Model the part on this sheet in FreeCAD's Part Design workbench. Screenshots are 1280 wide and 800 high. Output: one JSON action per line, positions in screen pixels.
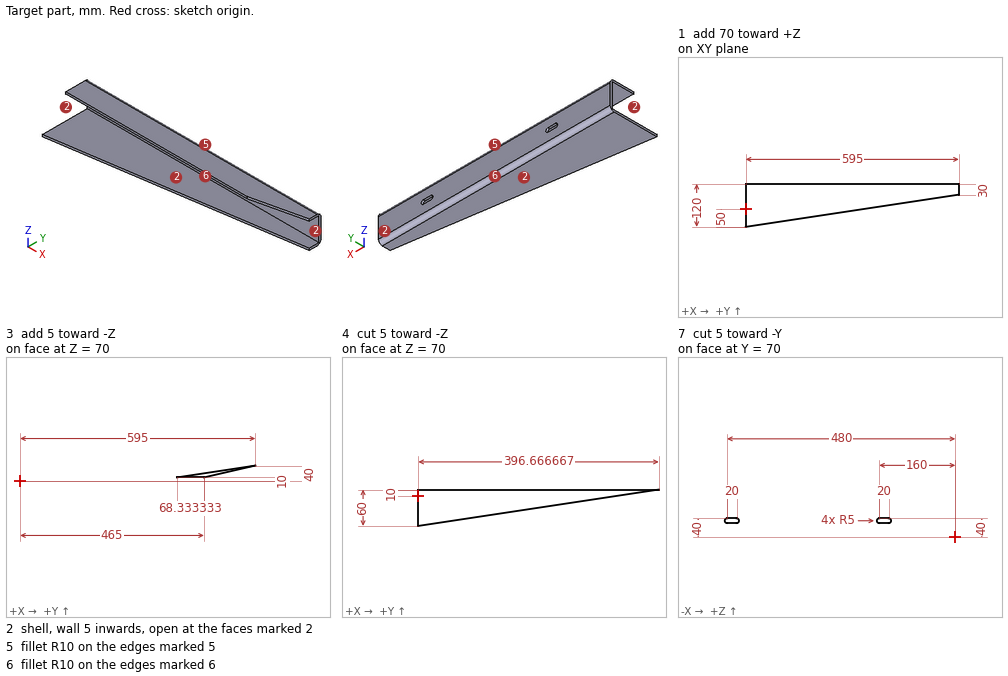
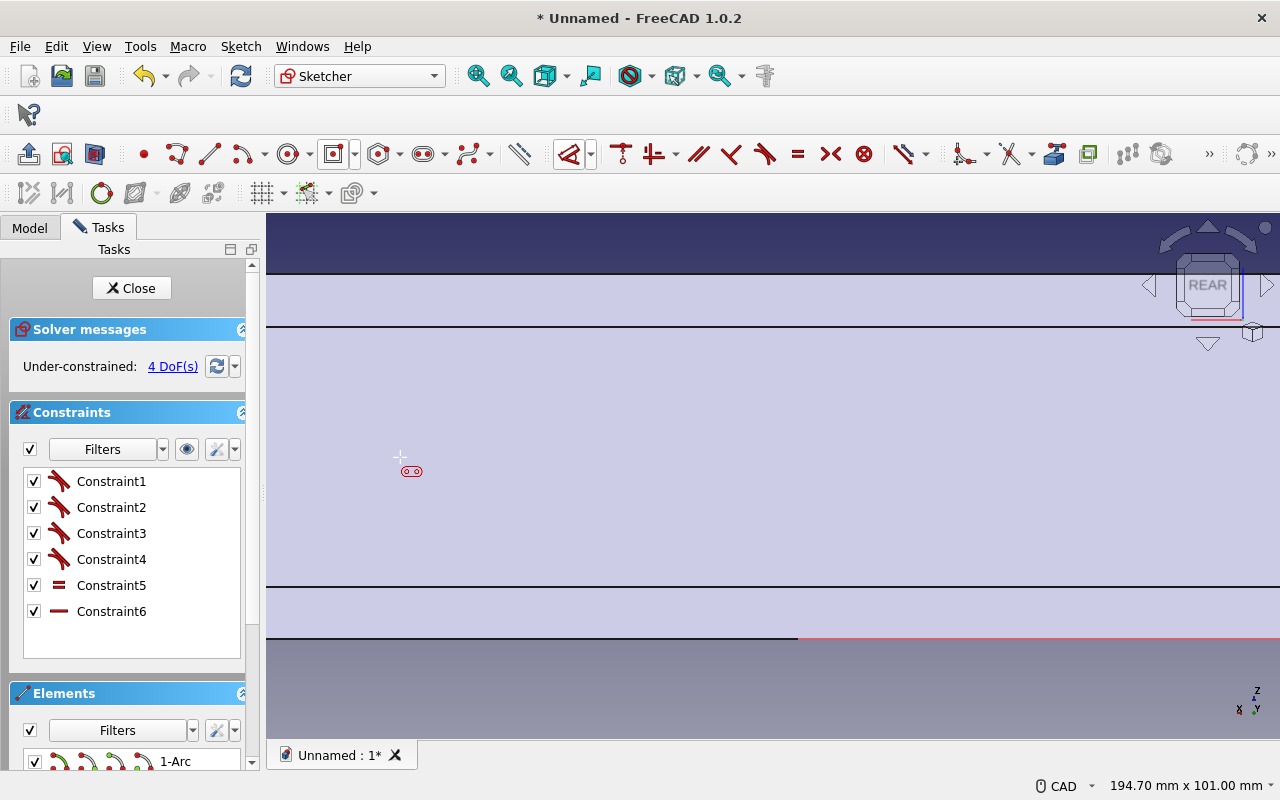
{"action": "scroll", "coordinate": [400, 457], "scroll_direction": "down", "scroll_amount": 7}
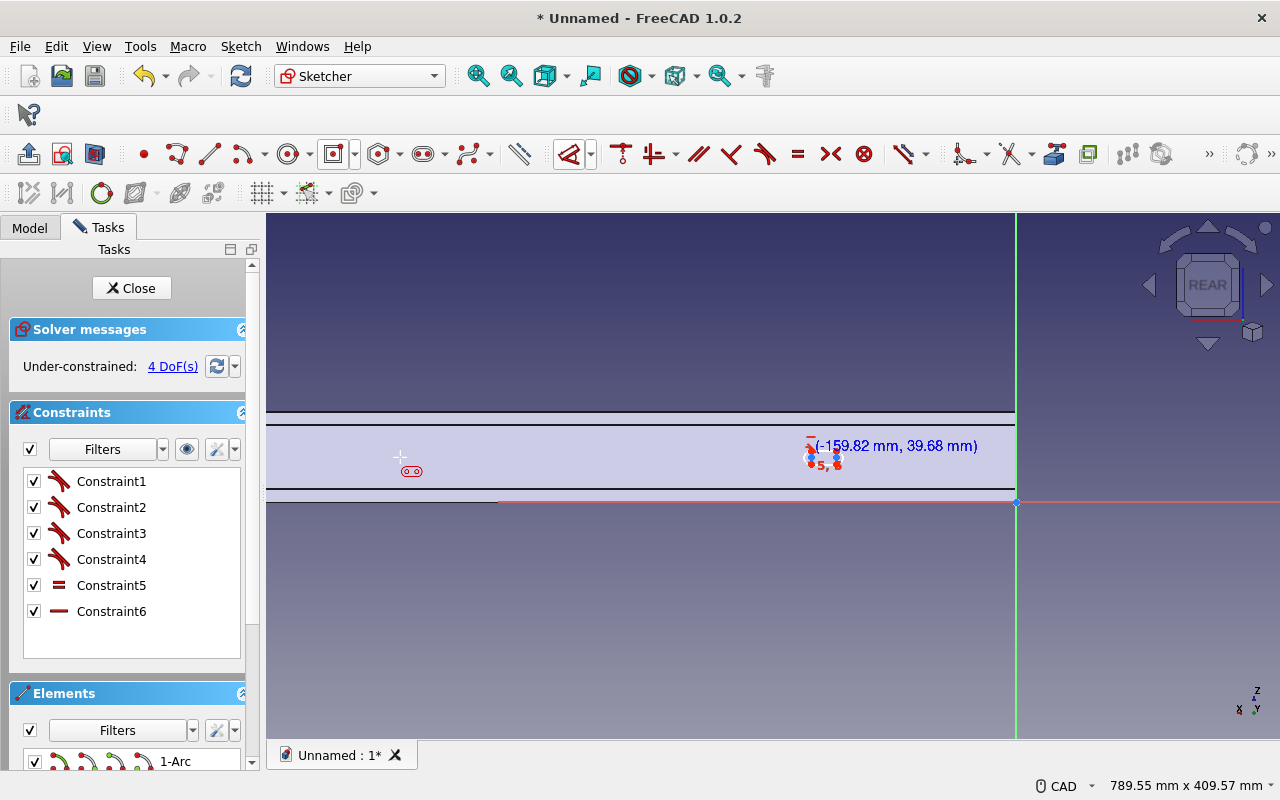
{"action": "left_click", "coordinate": [400, 457]}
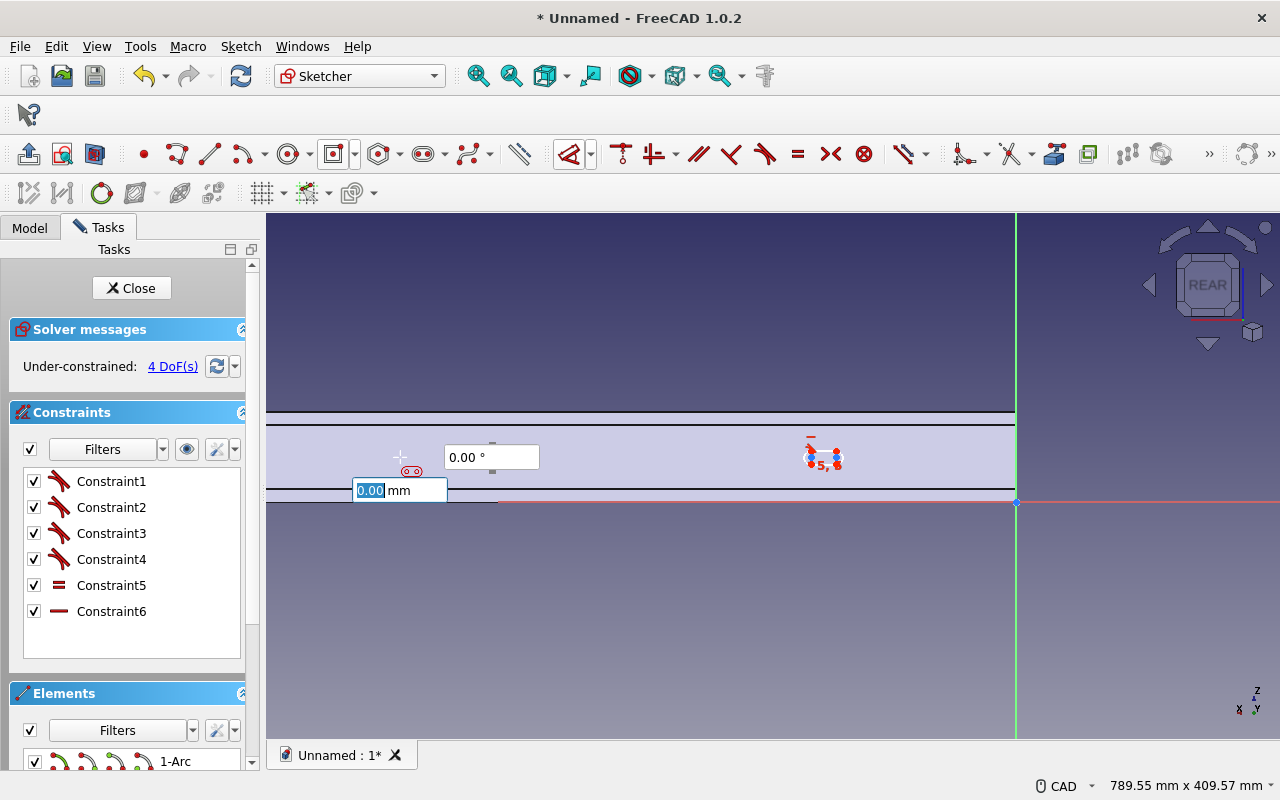
{"action": "left_click", "coordinate": [425, 457]}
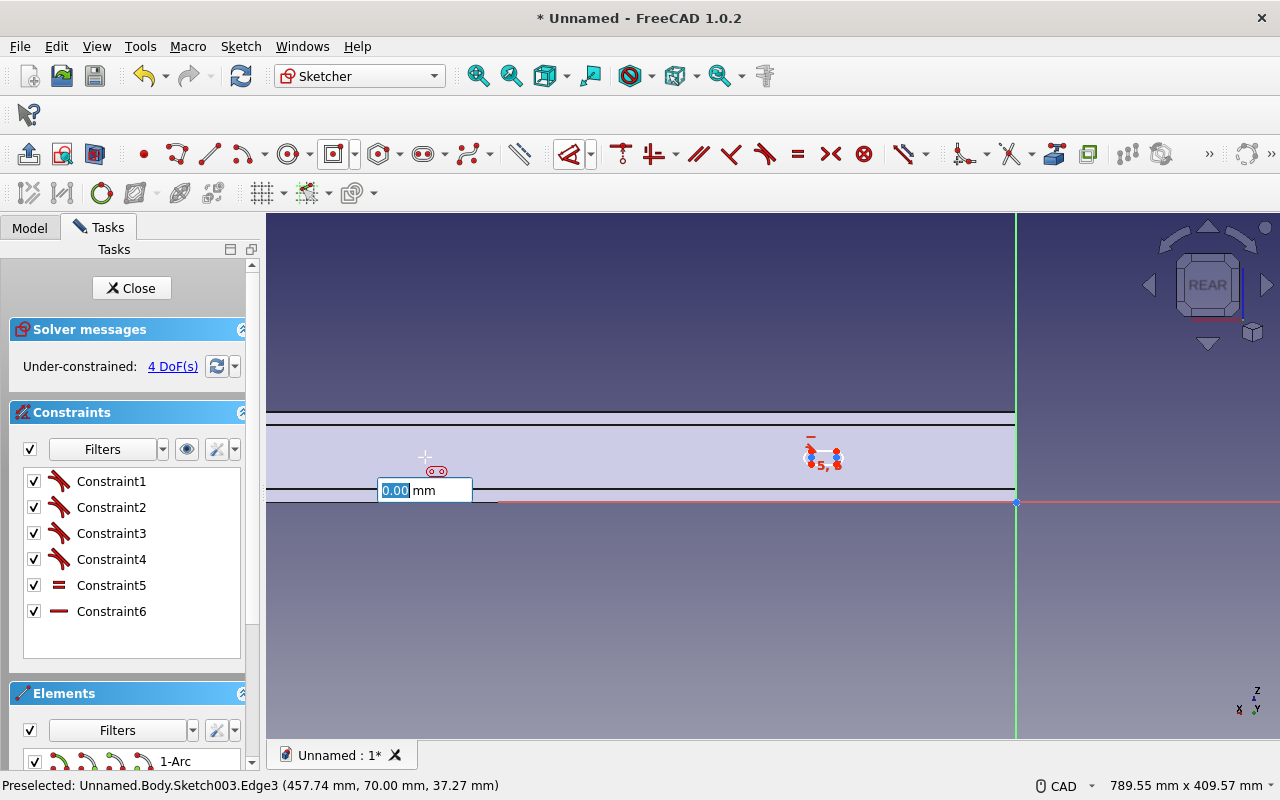
{"action": "scroll", "coordinate": [413, 464], "scroll_direction": "up", "scroll_amount": 5}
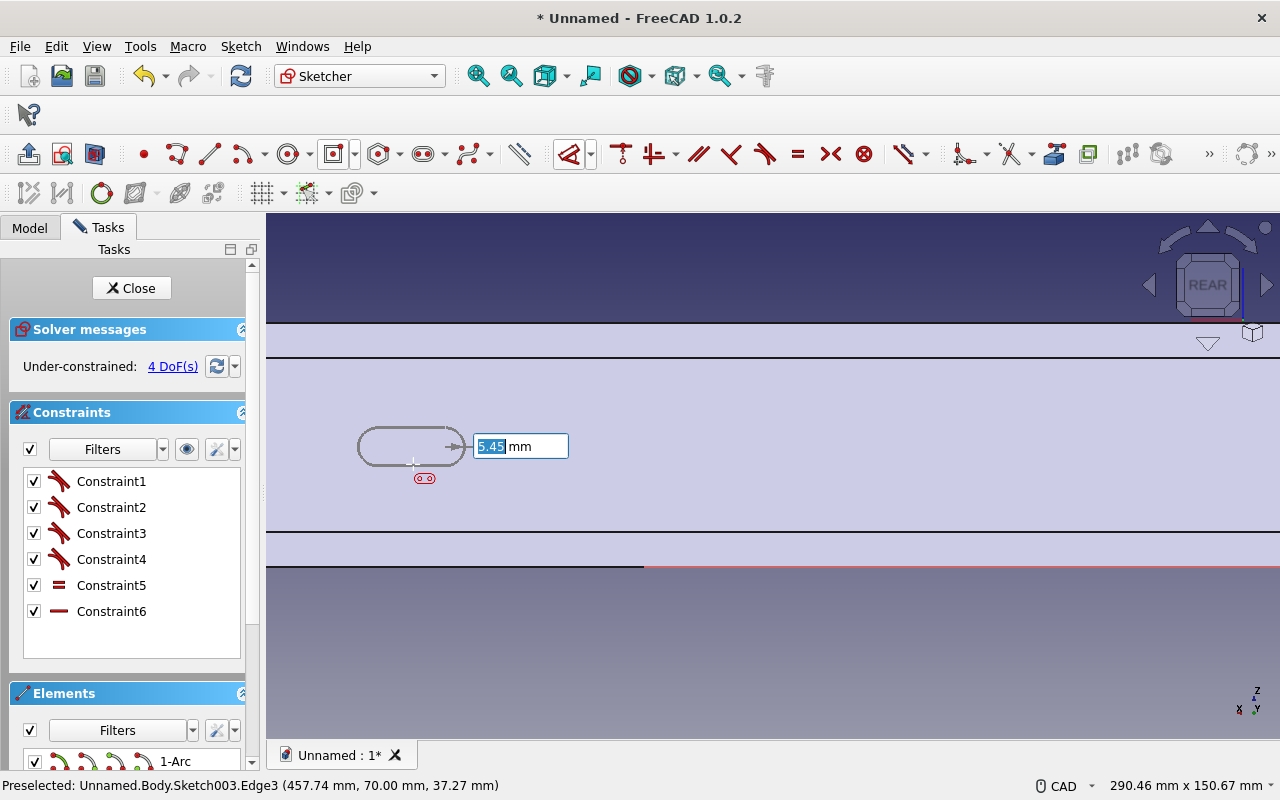
{"action": "left_click", "coordinate": [412, 462]}
{"action": "key", "text": "Escape"}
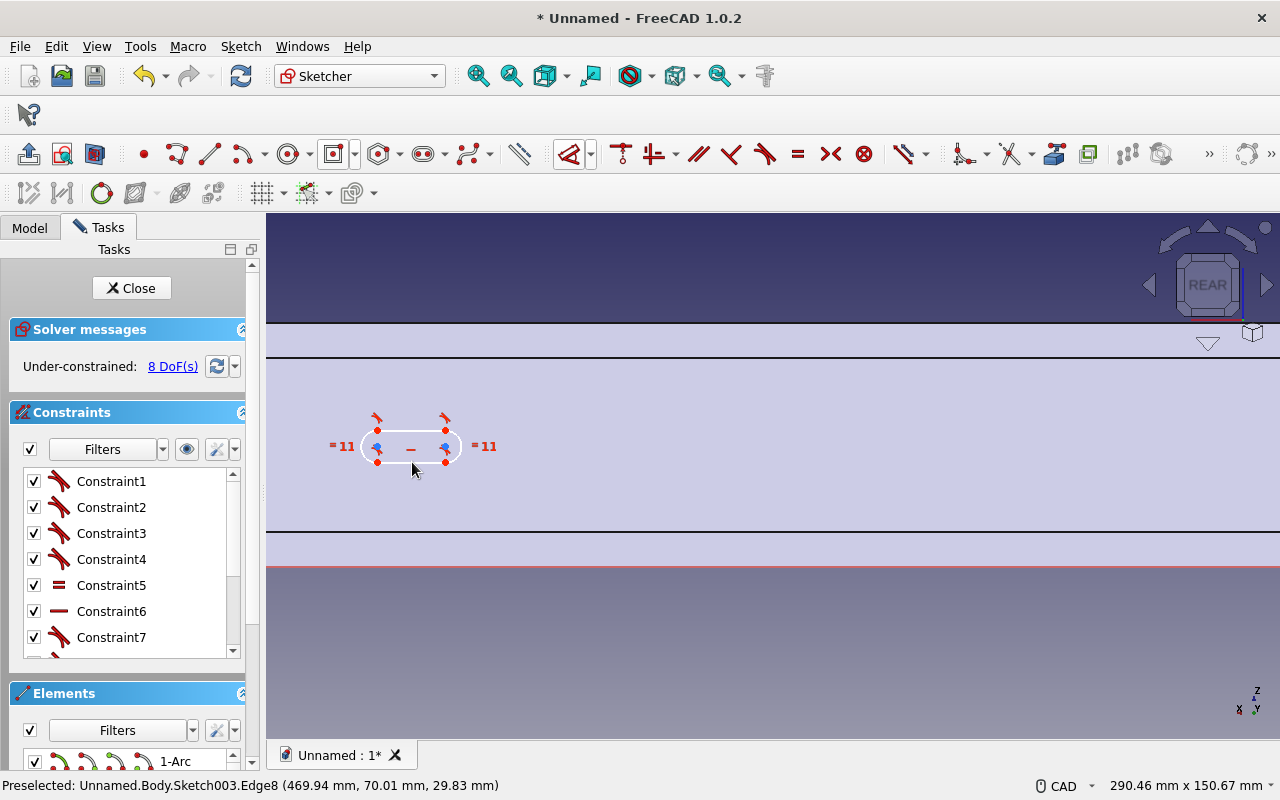
{"action": "scroll", "coordinate": [413, 464], "scroll_direction": "down", "scroll_amount": 5}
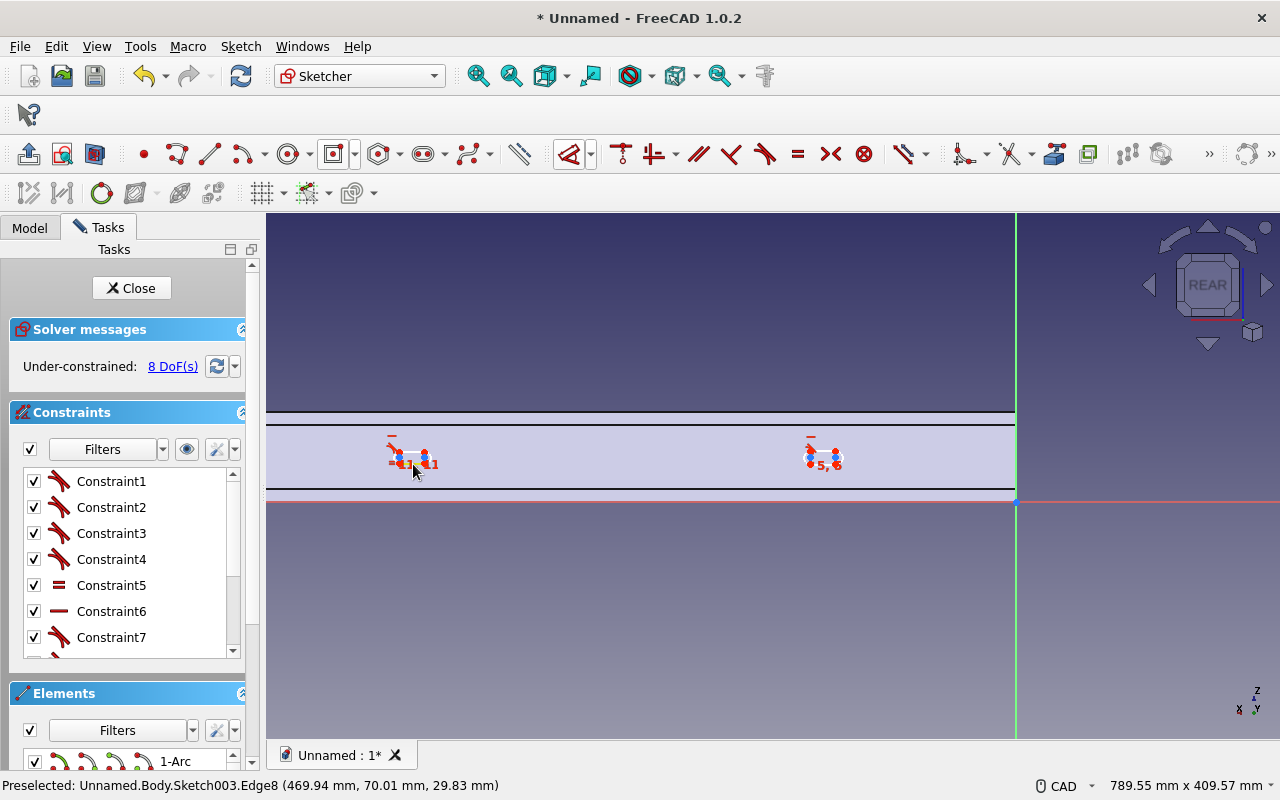
{"action": "scroll", "coordinate": [806, 454], "scroll_direction": "up", "scroll_amount": 5}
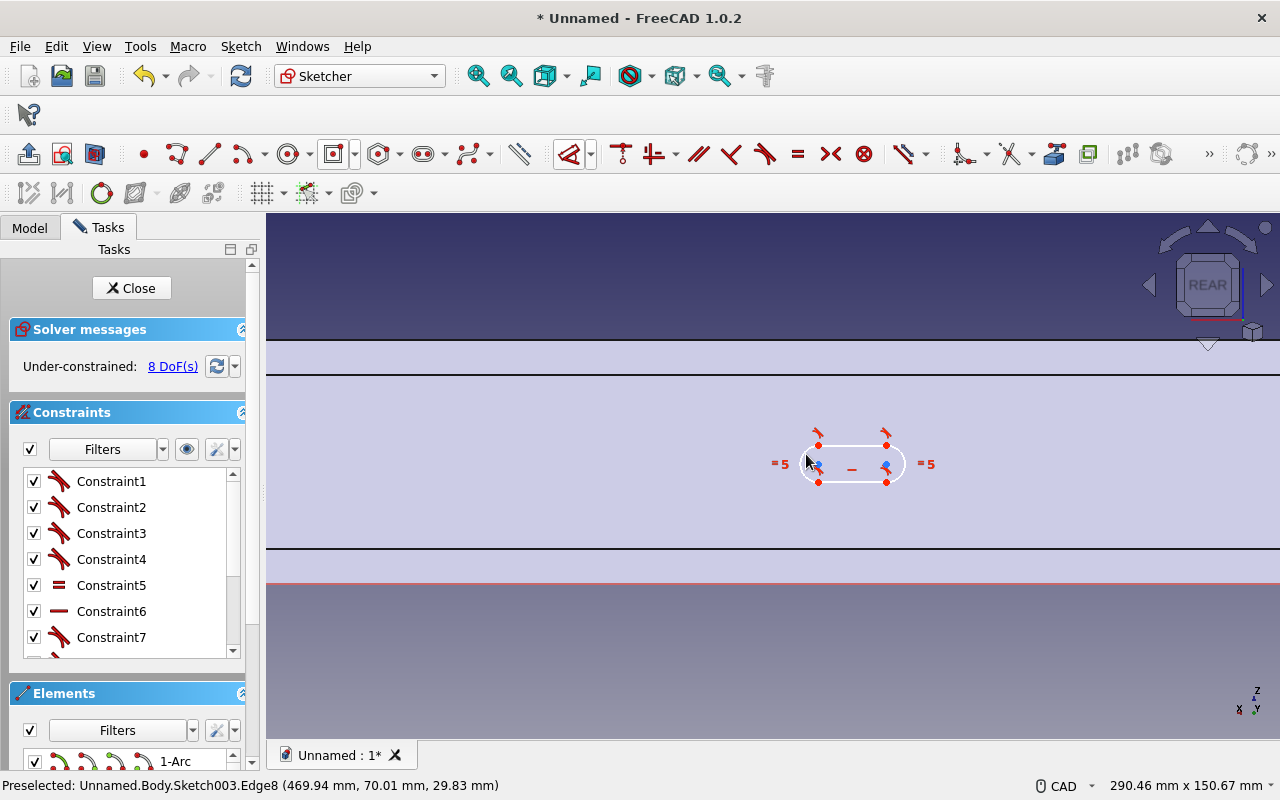
{"action": "left_click", "coordinate": [804, 453]}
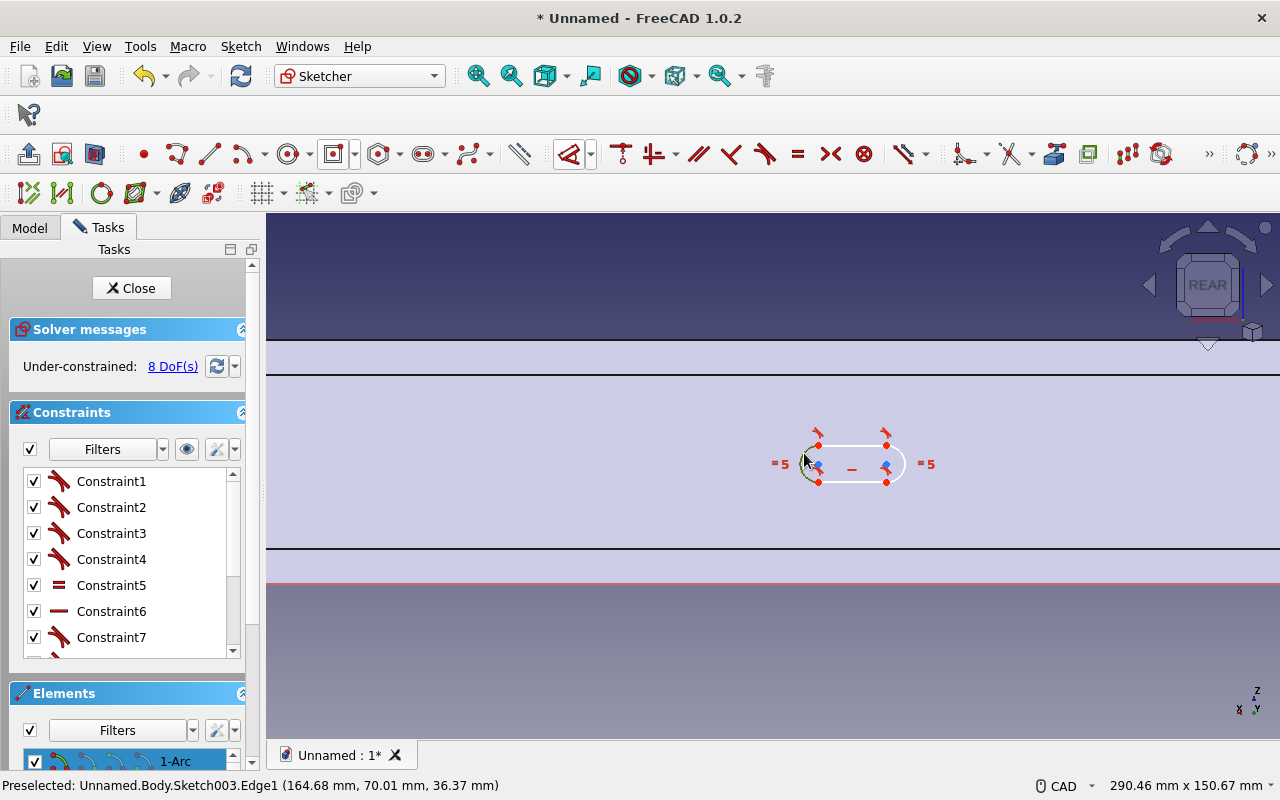
{"action": "scroll", "coordinate": [806, 454], "scroll_direction": "down", "scroll_amount": 5}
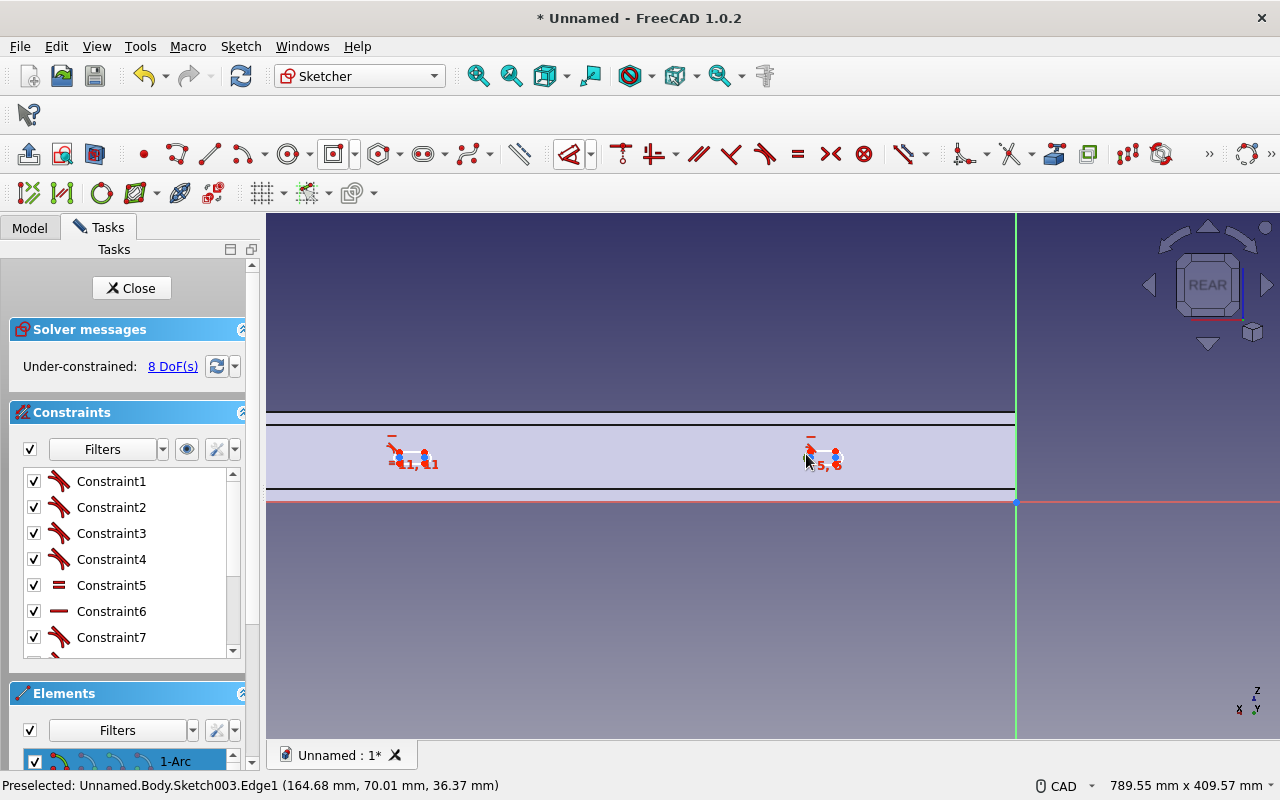
{"action": "scroll", "coordinate": [395, 455], "scroll_direction": "up", "scroll_amount": 5}